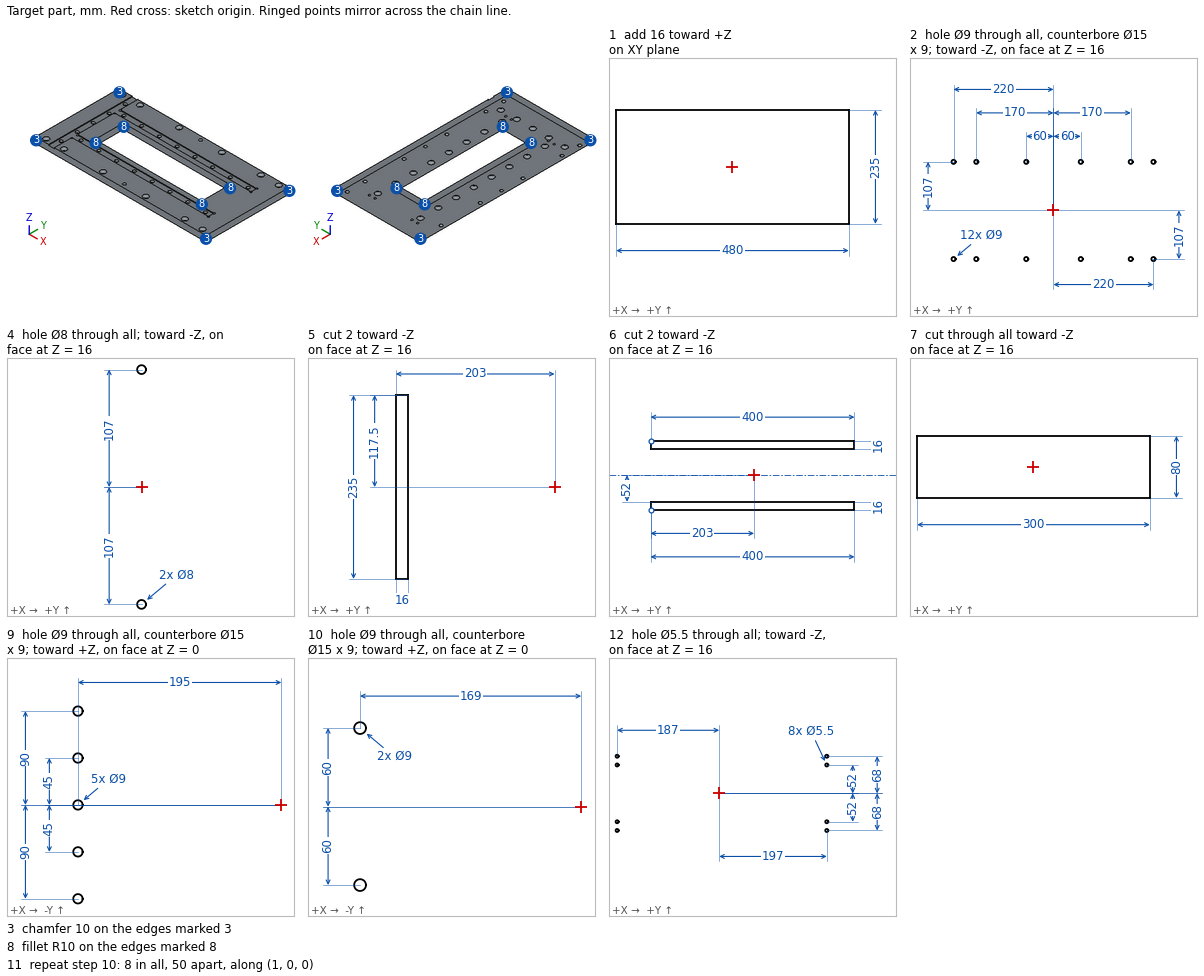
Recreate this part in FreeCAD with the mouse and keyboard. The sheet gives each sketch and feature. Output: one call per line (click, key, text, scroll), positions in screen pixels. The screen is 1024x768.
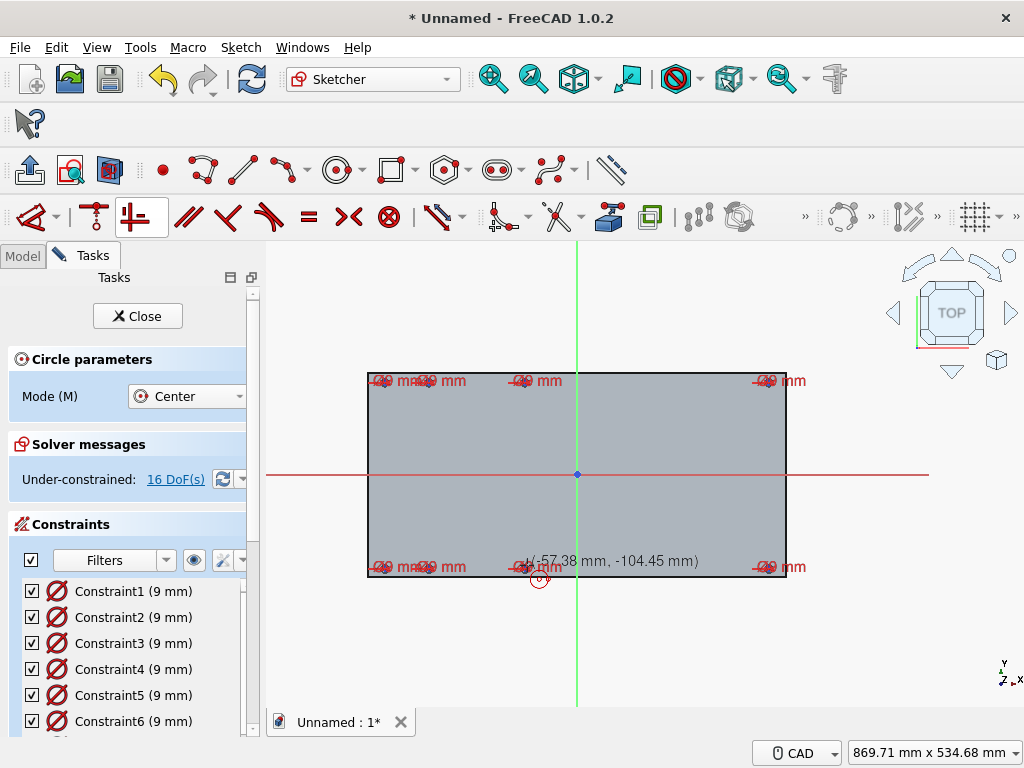
scroll(629, 382, up, 9)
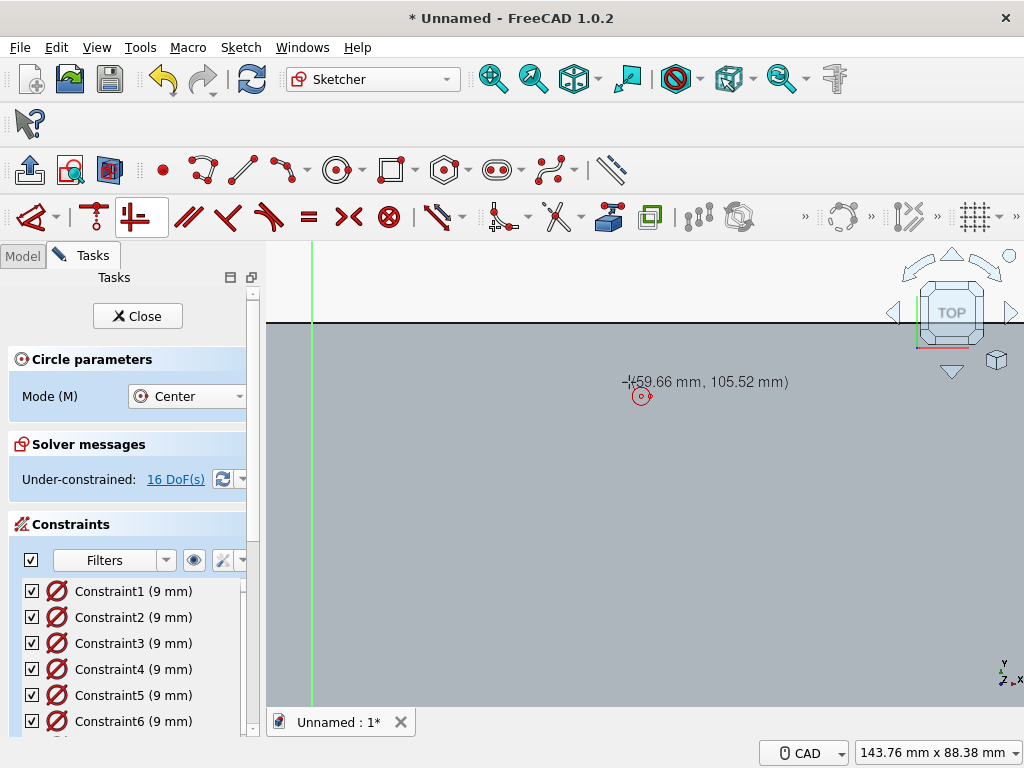
scroll(629, 381, down, 9)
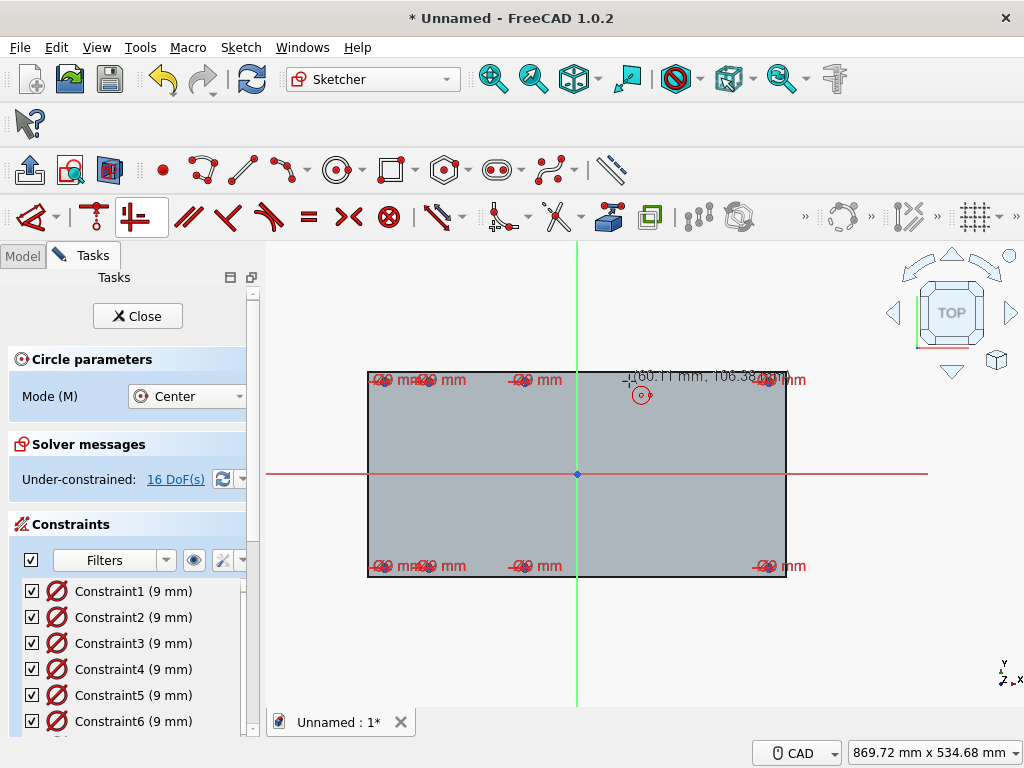
click(629, 381)
move(632, 378)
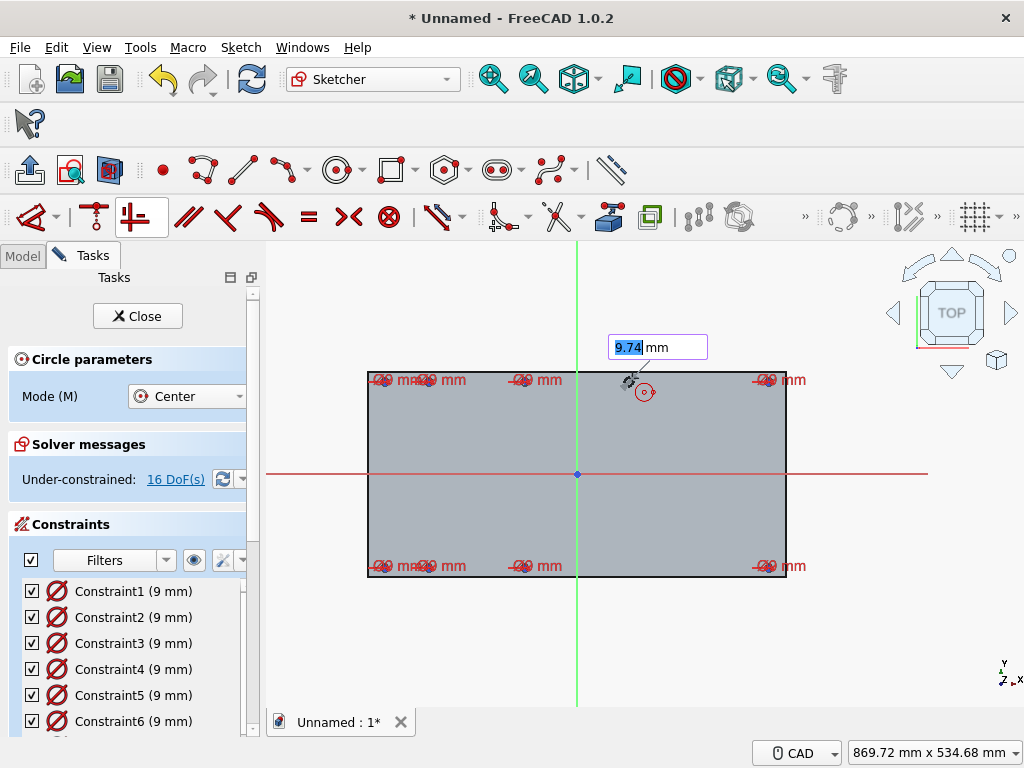
text(9)
key(Return)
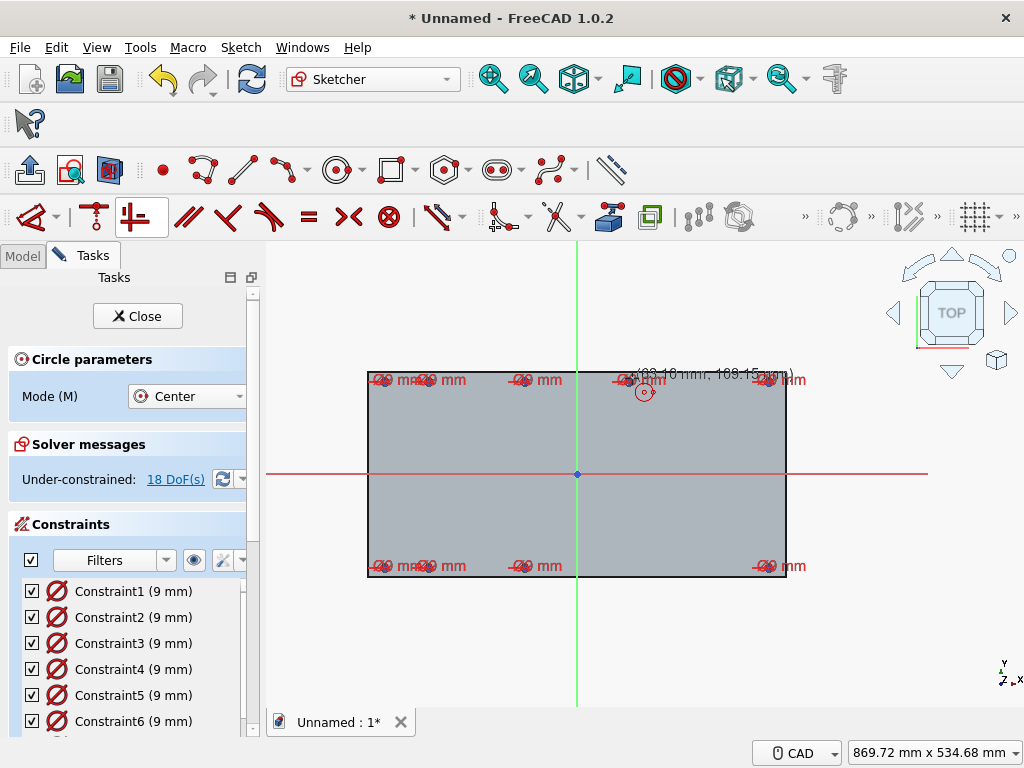
scroll(629, 567, up, 9)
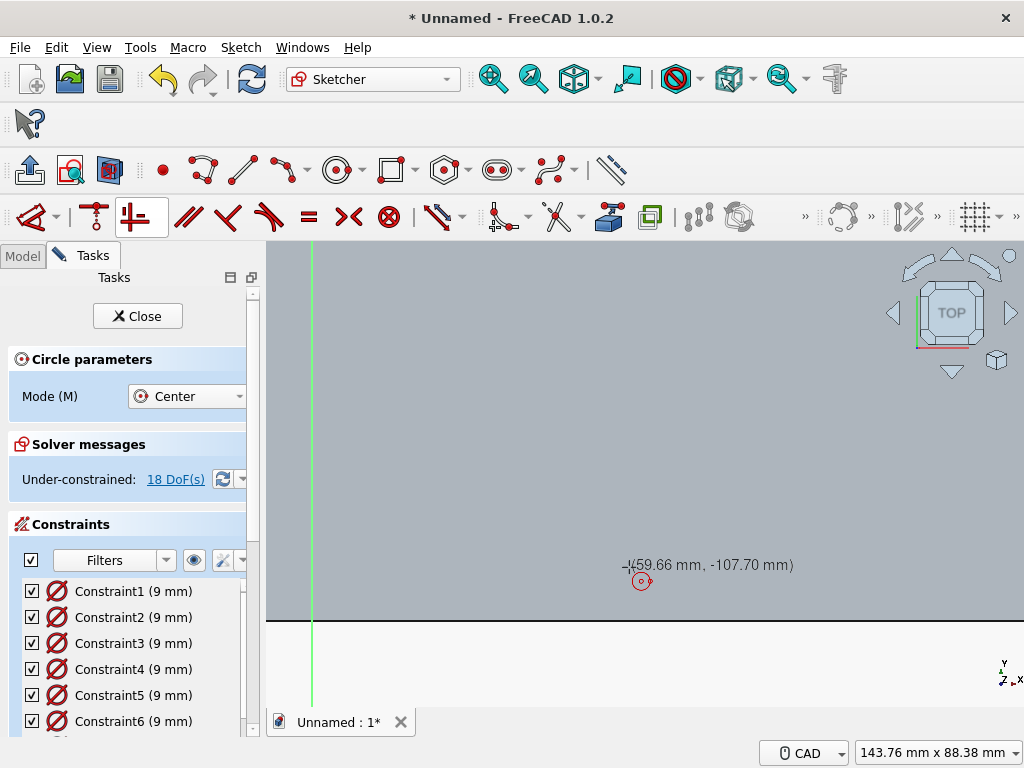
scroll(629, 568, down, 9)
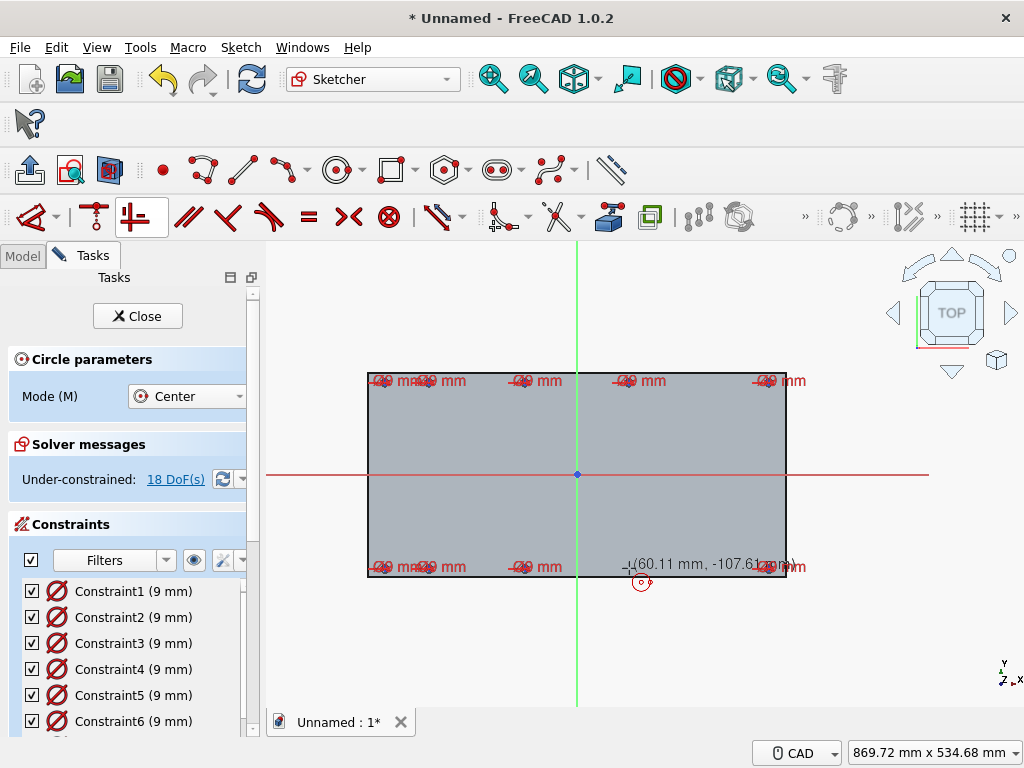
click(629, 568)
move(632, 565)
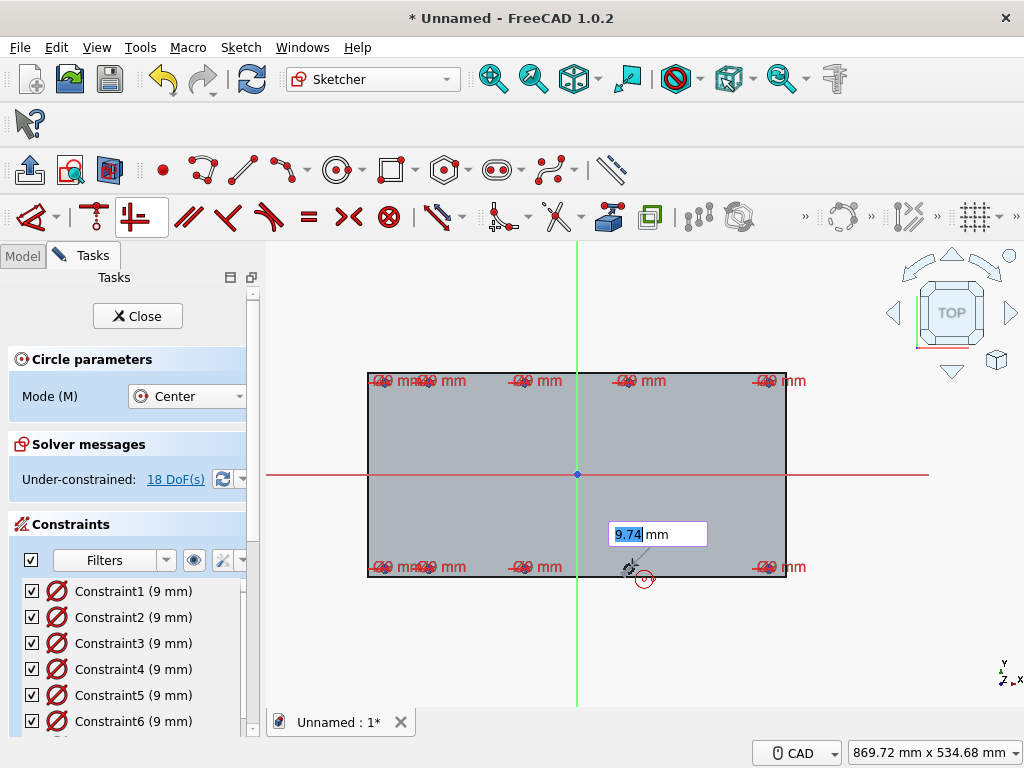
text(9)
key(Return)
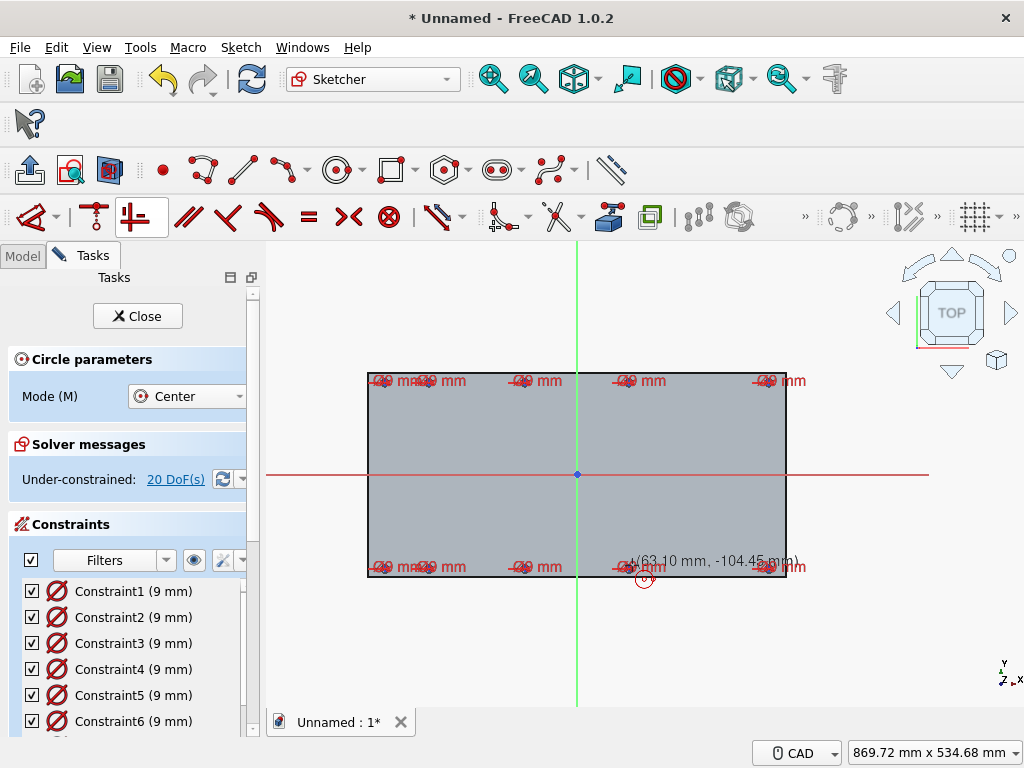
scroll(725, 382, up, 9)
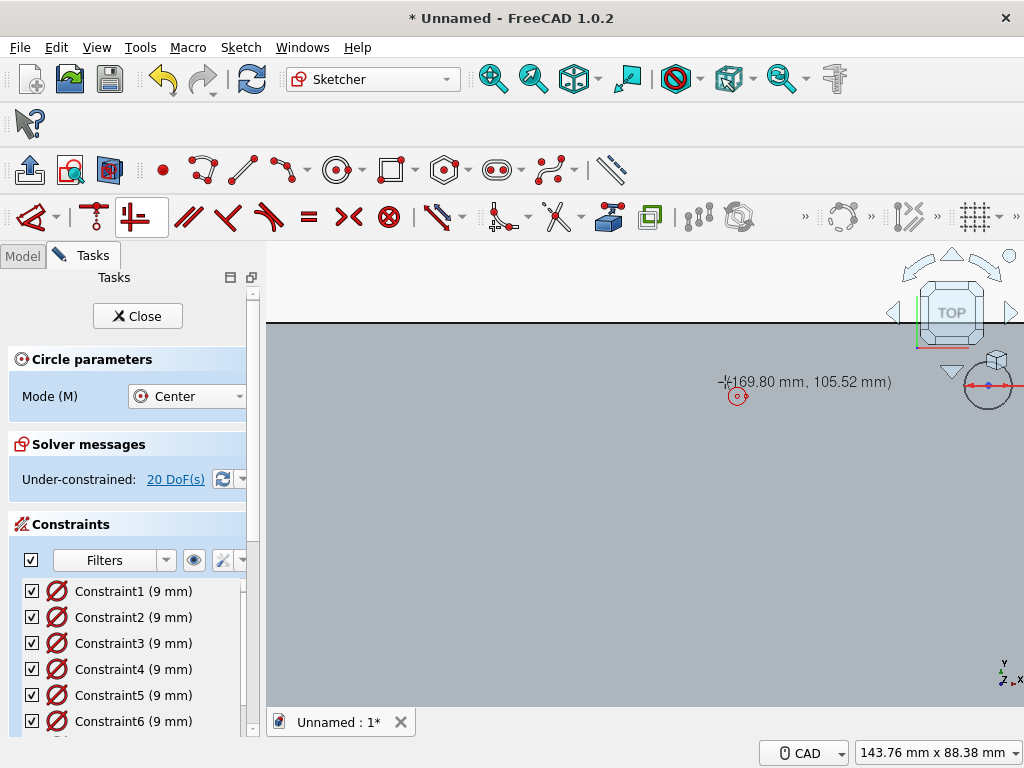
scroll(725, 381, down, 9)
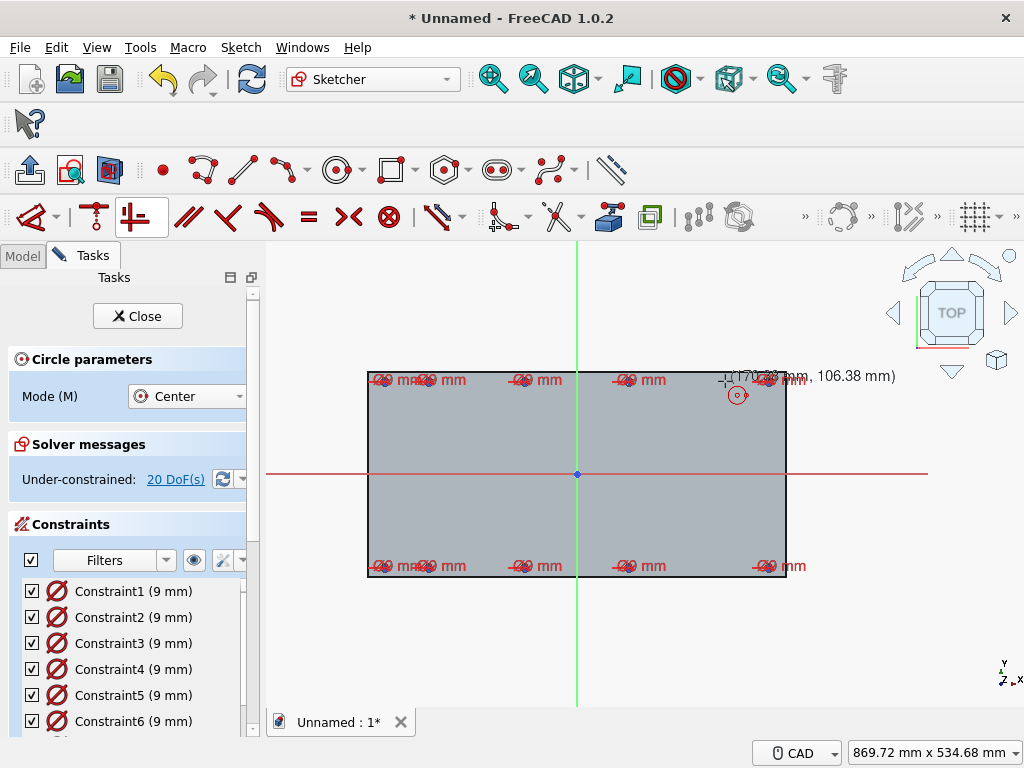
click(725, 381)
move(728, 378)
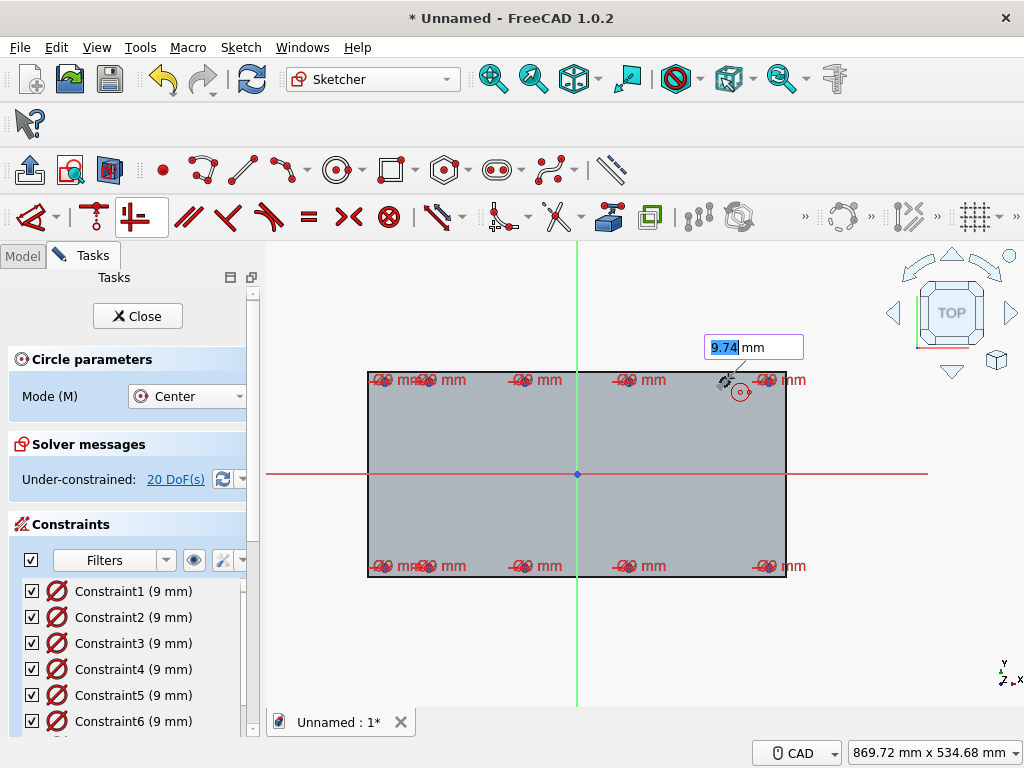
text(9)
key(Return)